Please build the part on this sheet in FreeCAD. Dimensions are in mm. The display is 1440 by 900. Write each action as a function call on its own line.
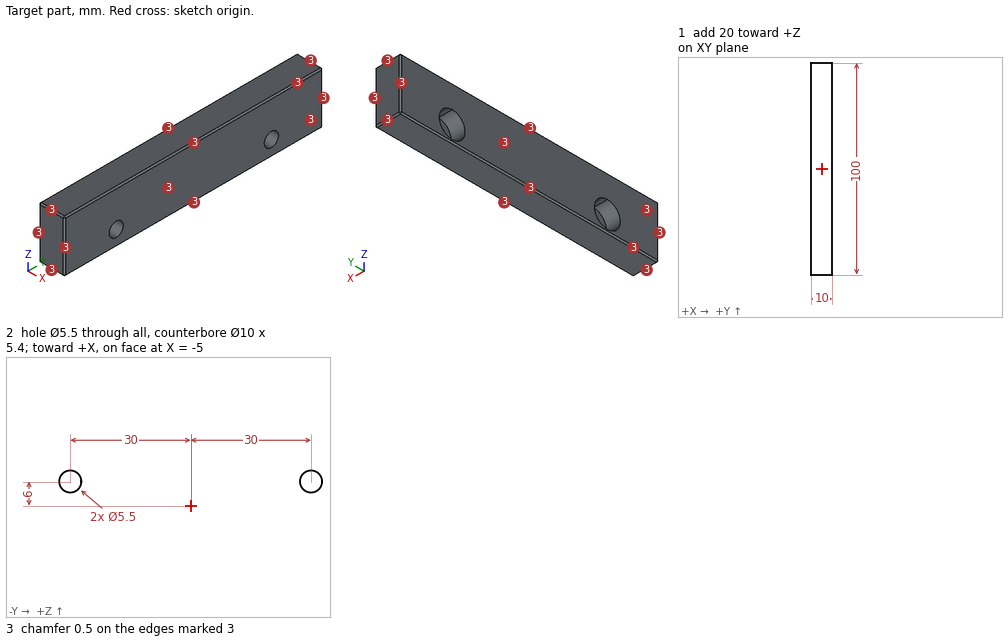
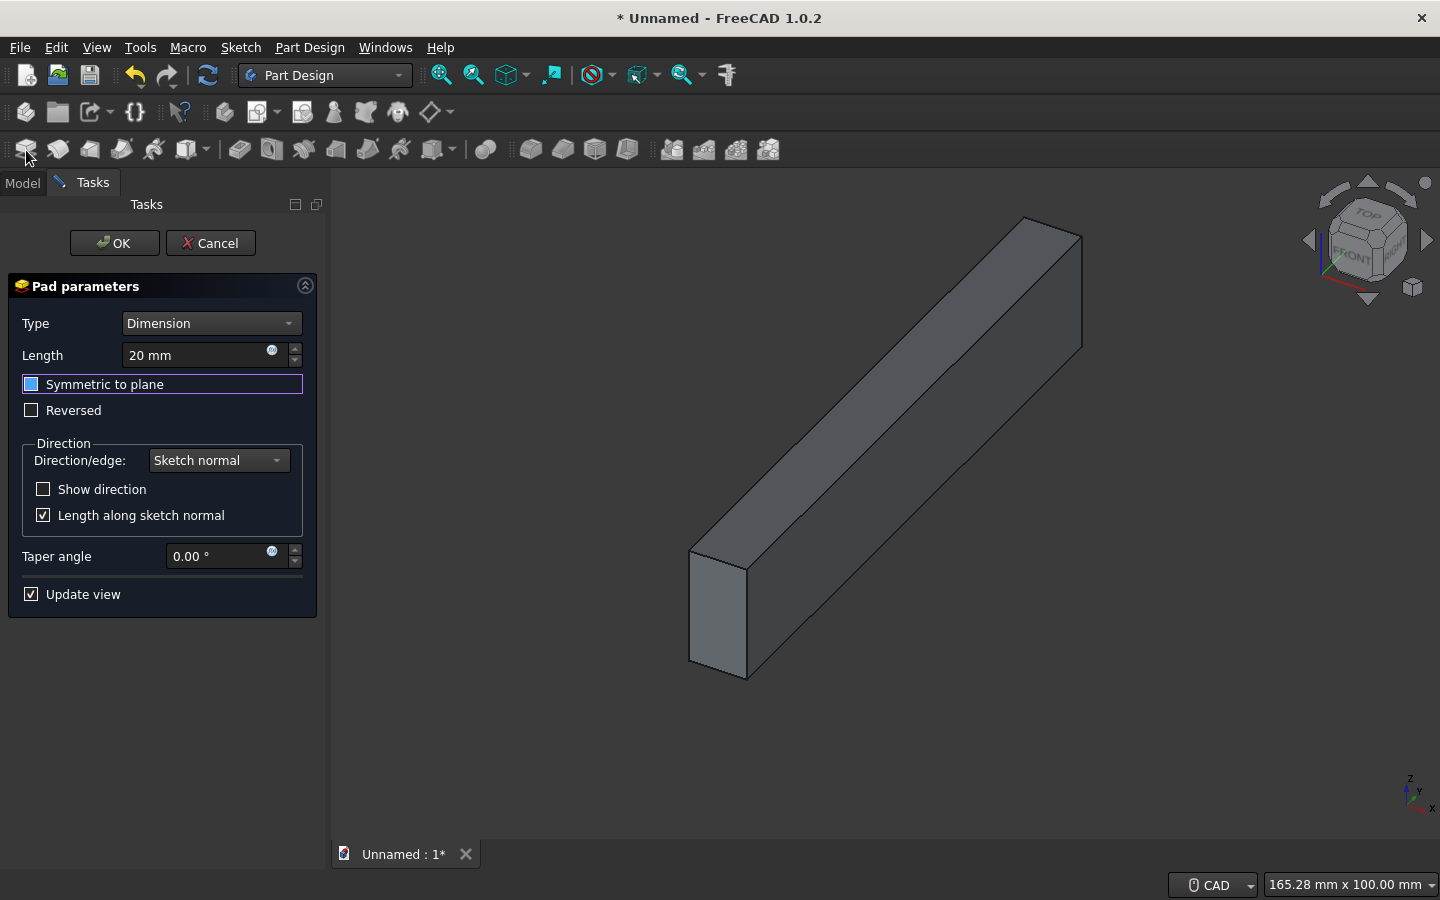
click(115, 243)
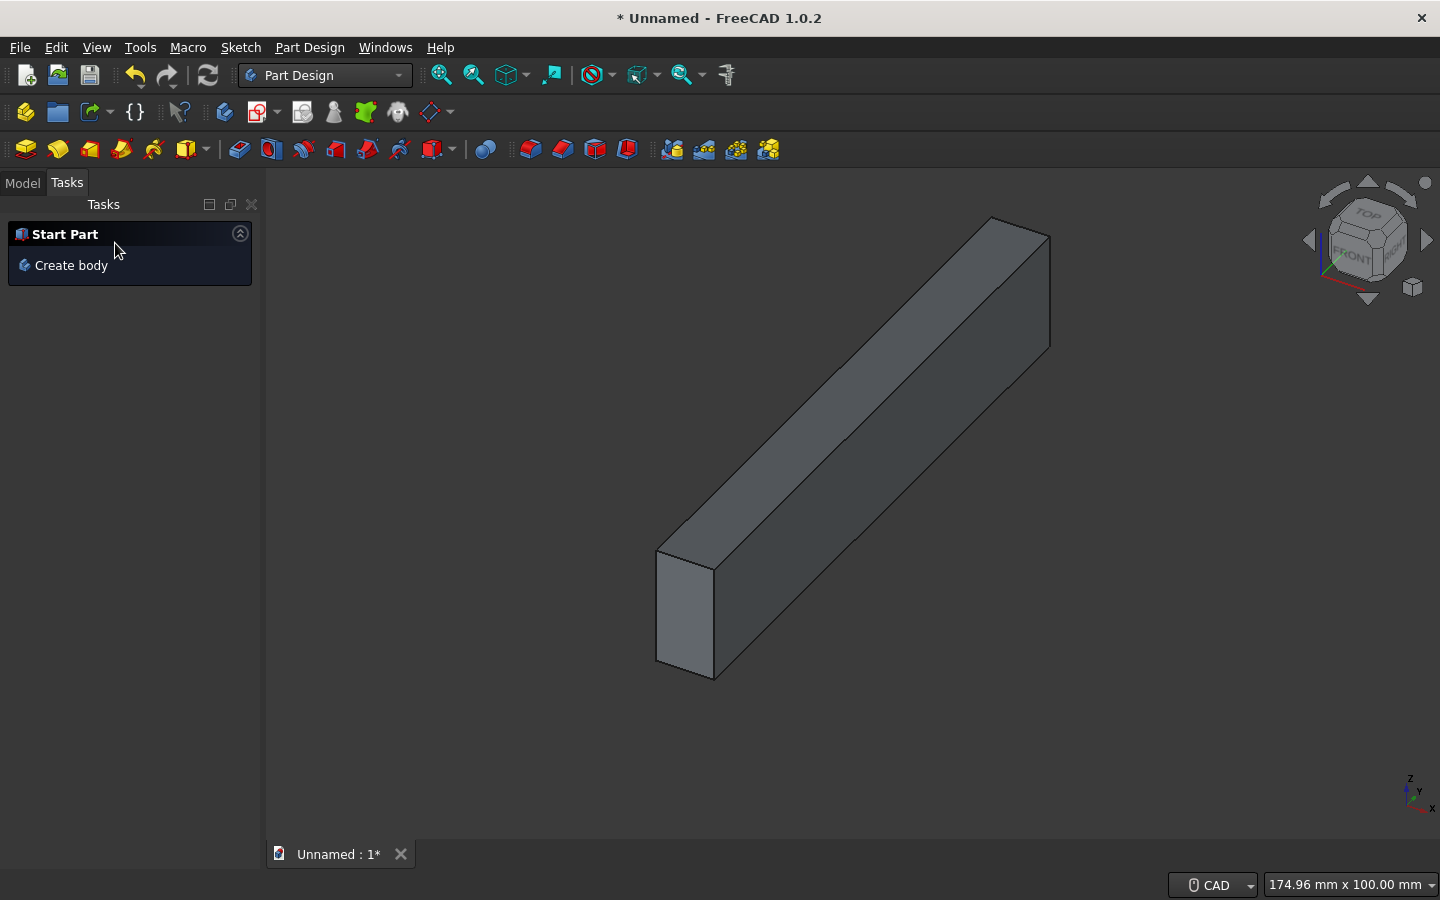
key(6)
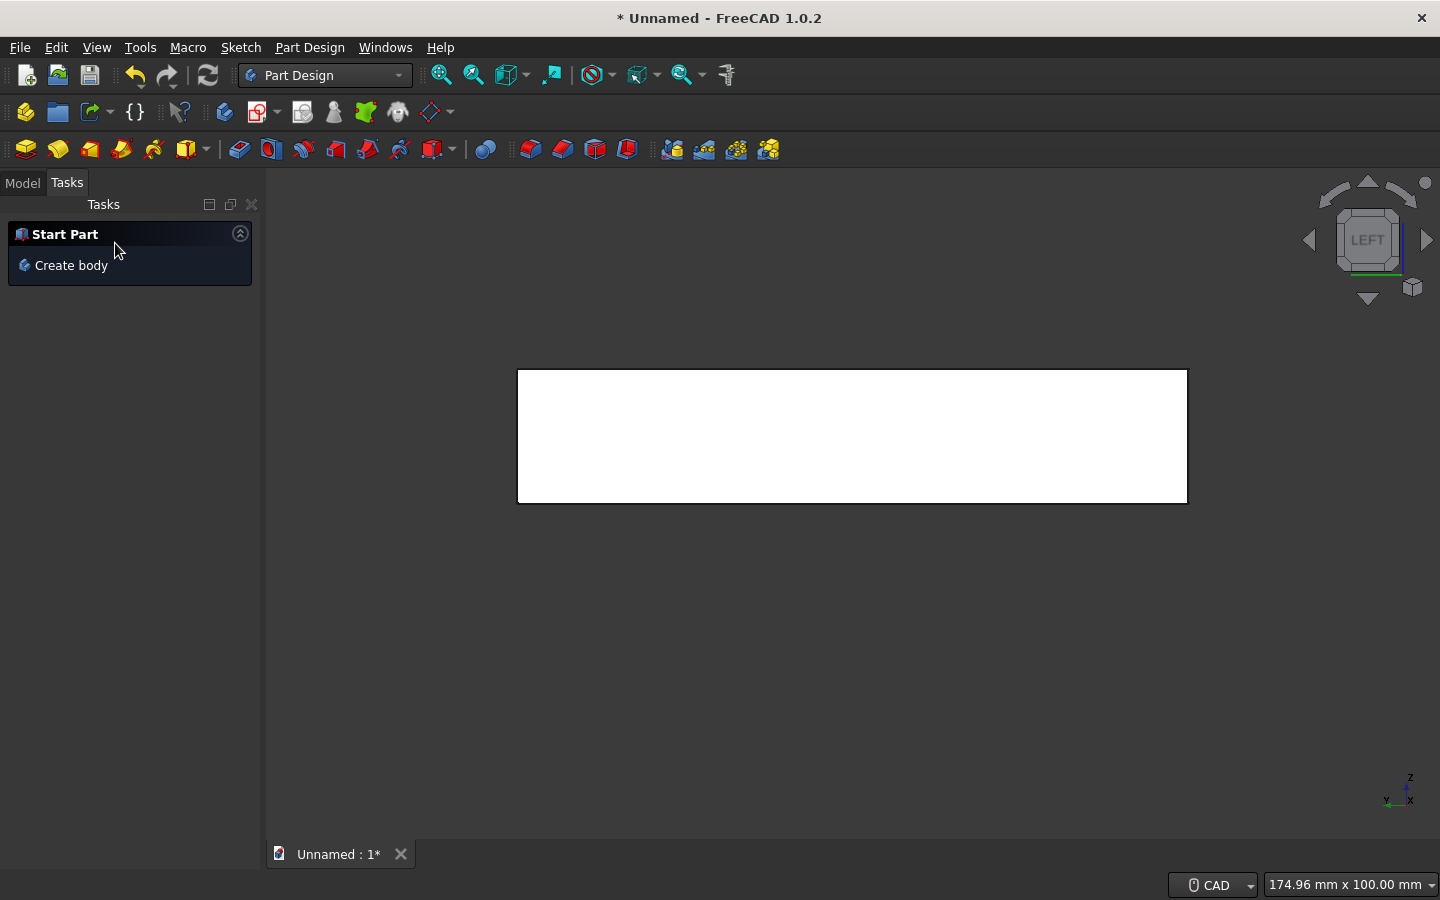
click(661, 435)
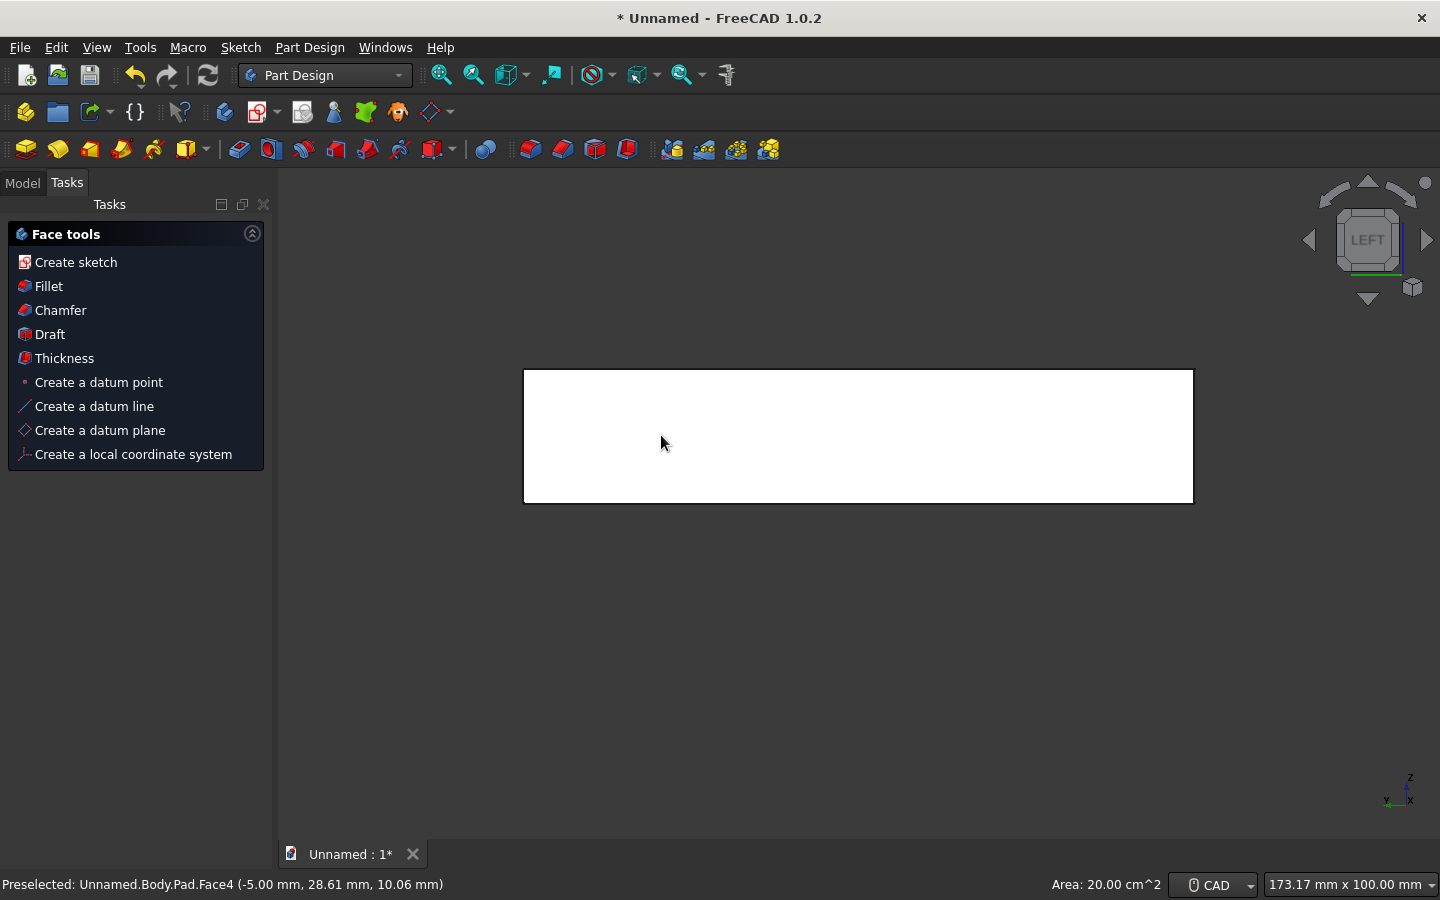
click(258, 112)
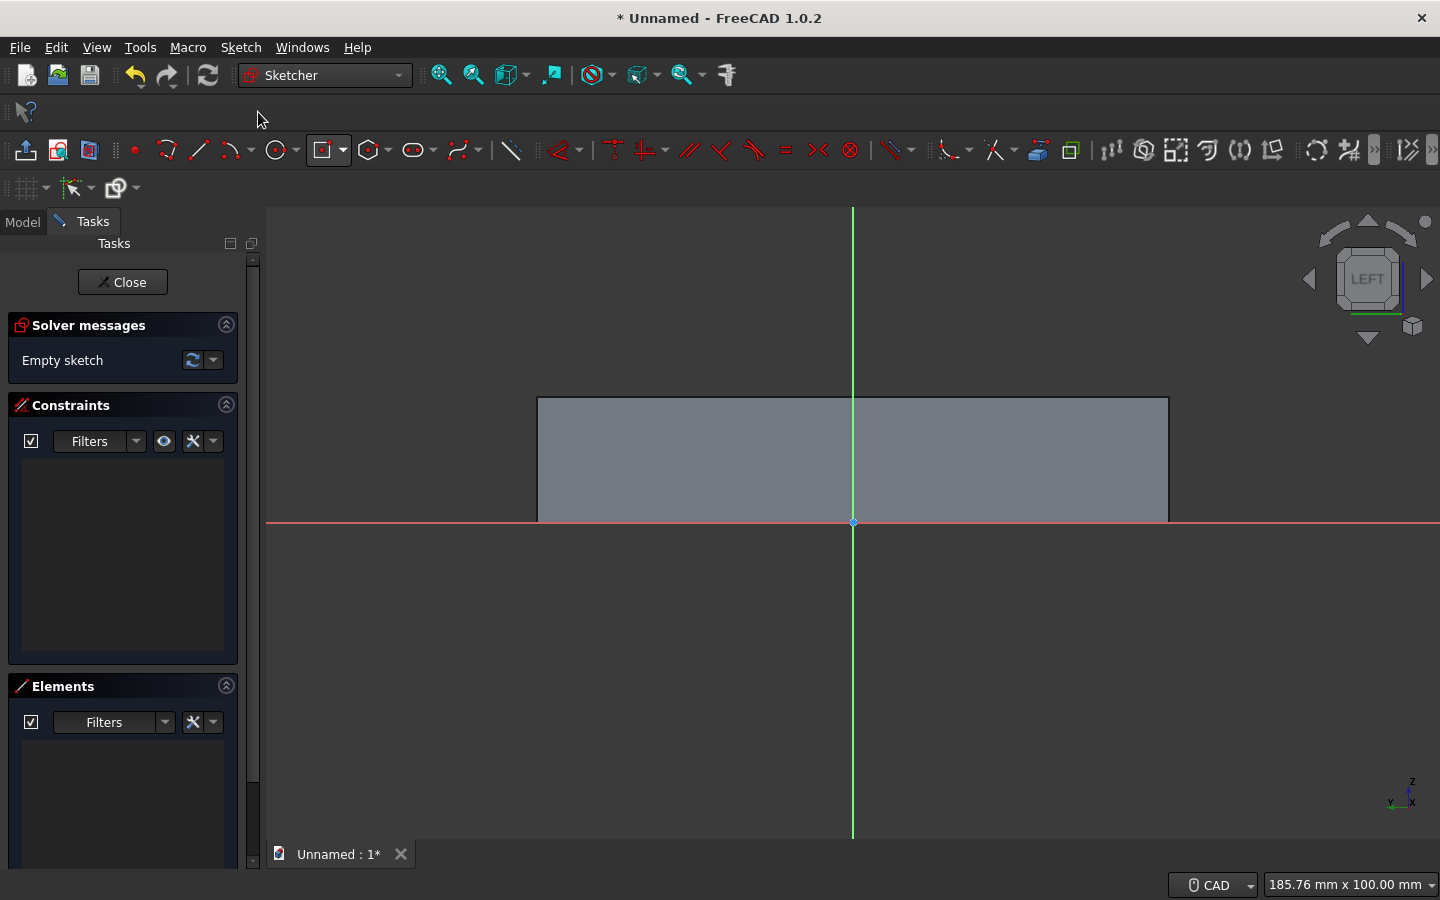
scroll(936, 462, up, 3)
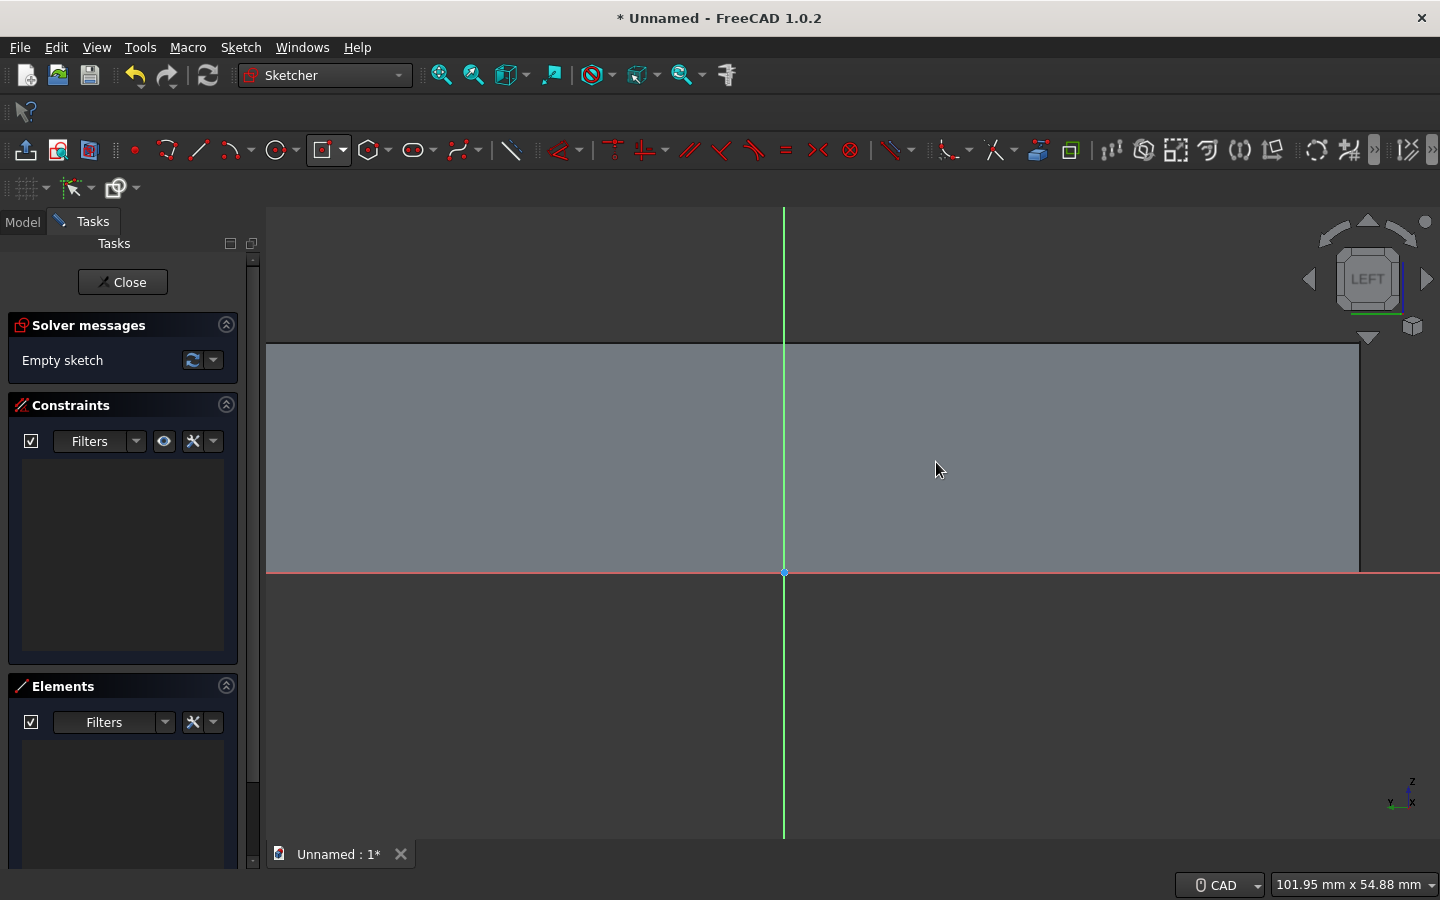
click(276, 150)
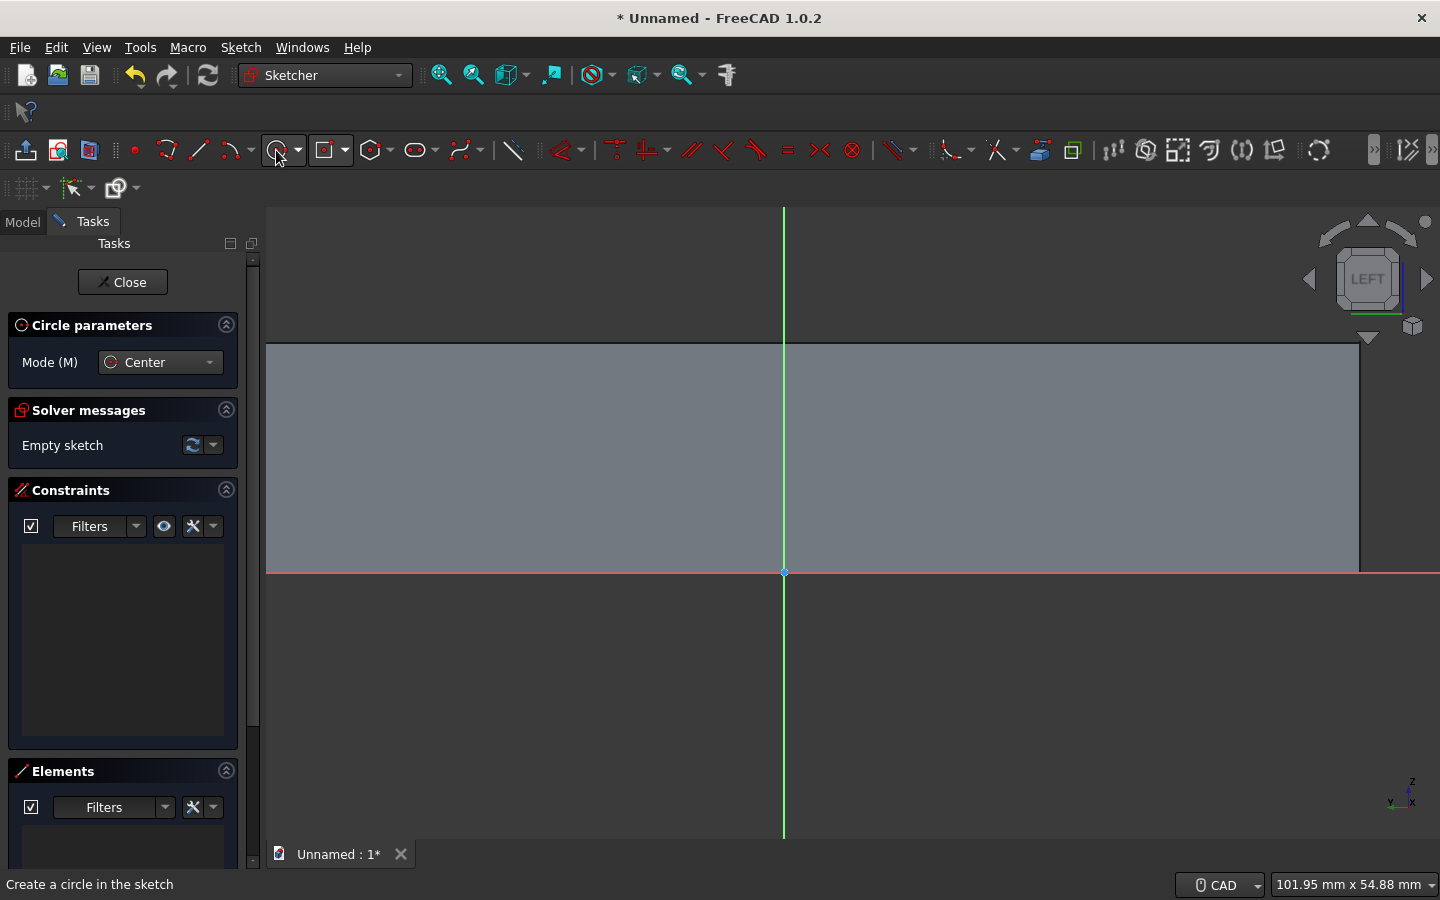
click(439, 504)
click(461, 481)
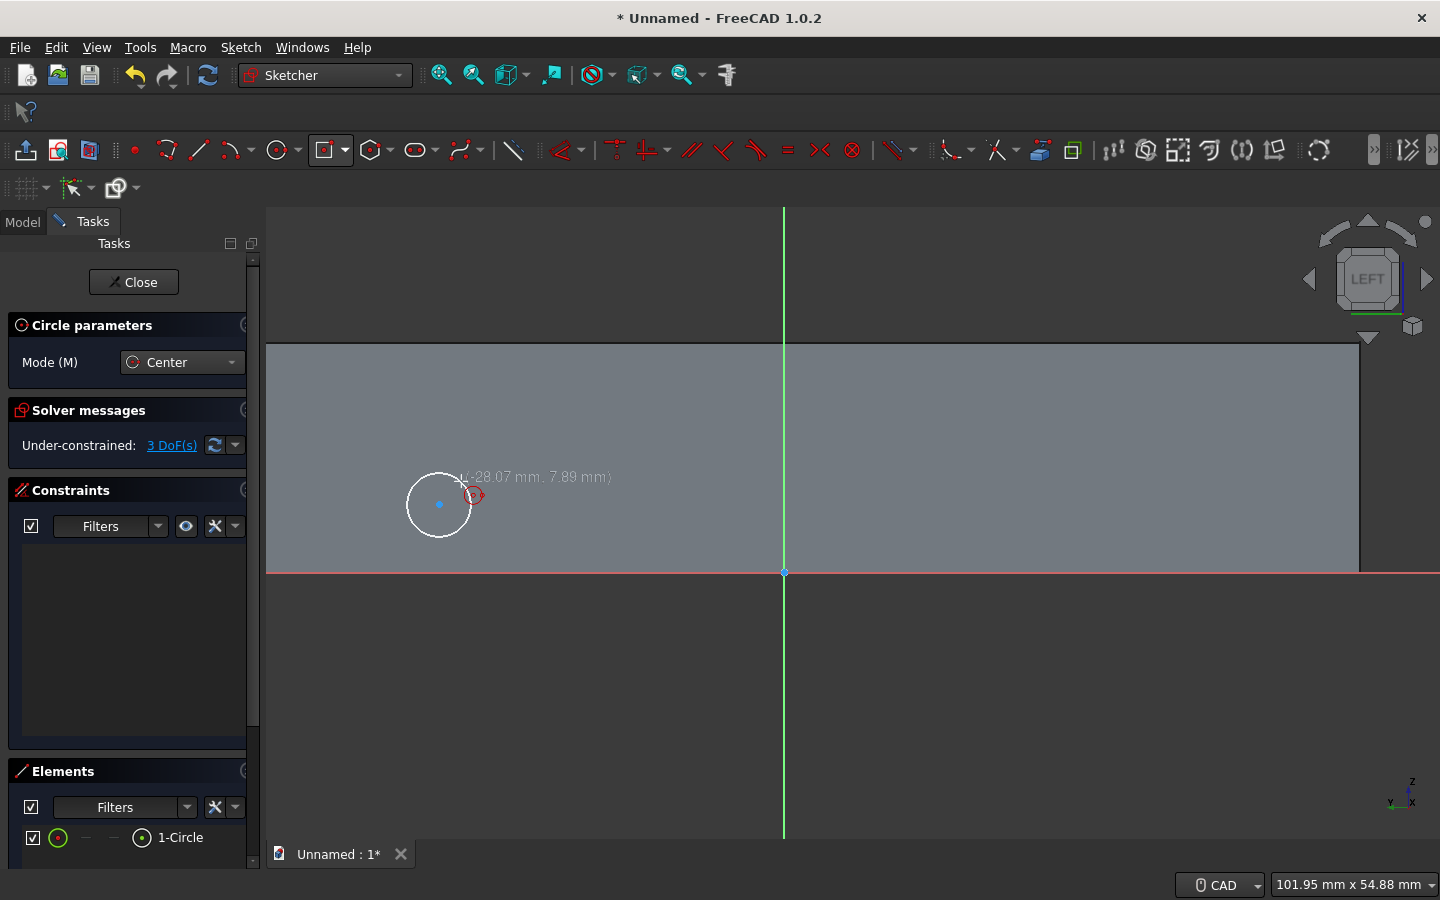
click(1130, 504)
click(1152, 481)
key(Escape)